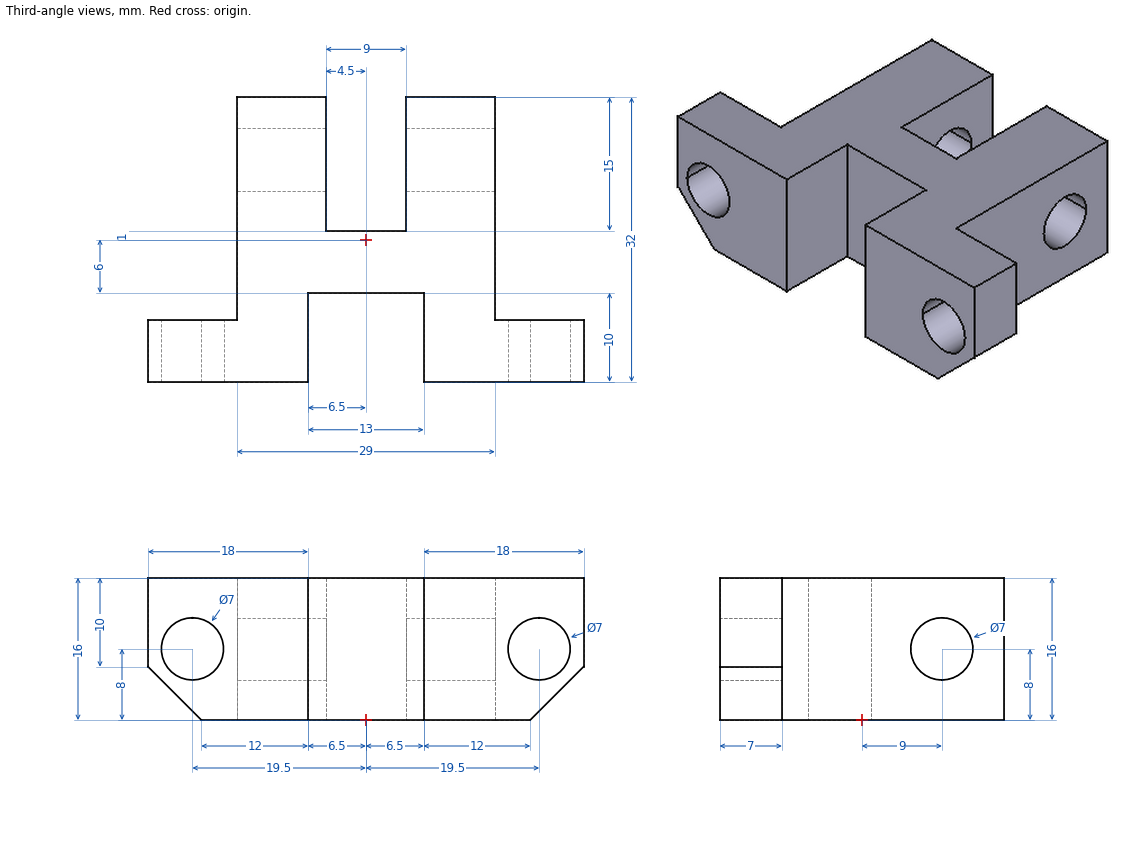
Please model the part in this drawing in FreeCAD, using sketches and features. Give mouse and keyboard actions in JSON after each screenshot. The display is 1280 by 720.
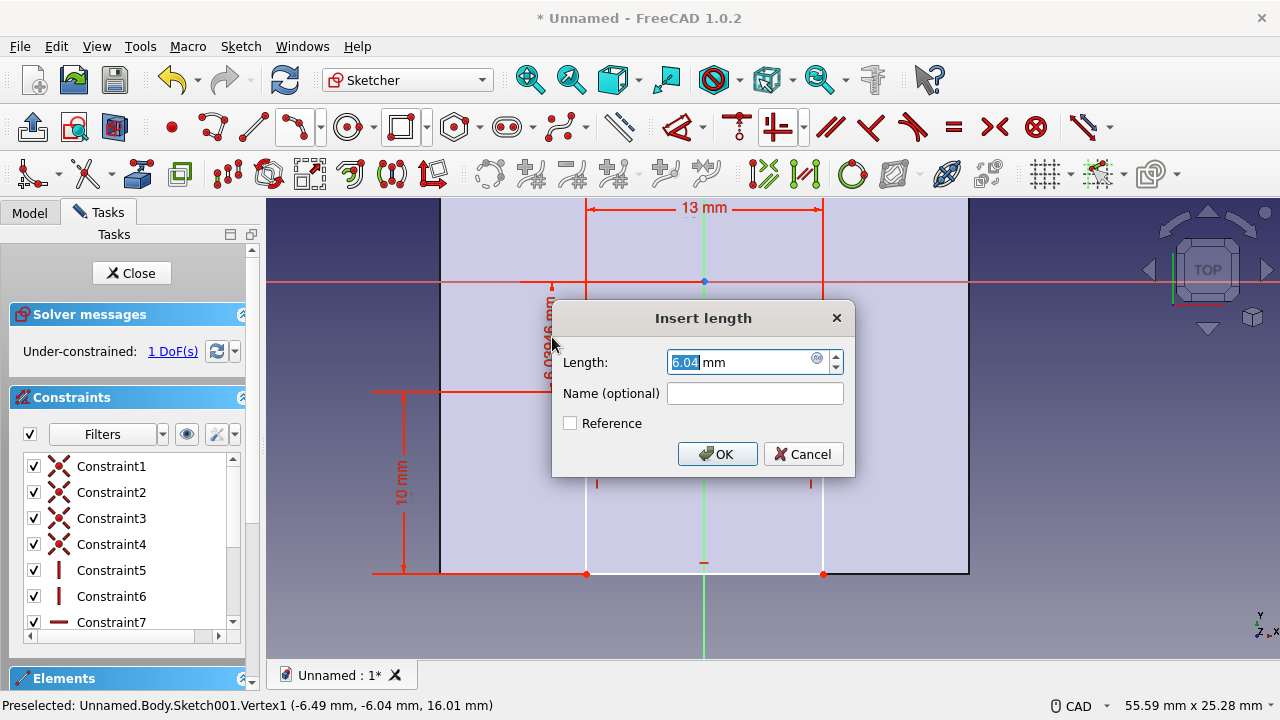
{"action": "type", "text": "6"}
{"action": "key", "text": "Return"}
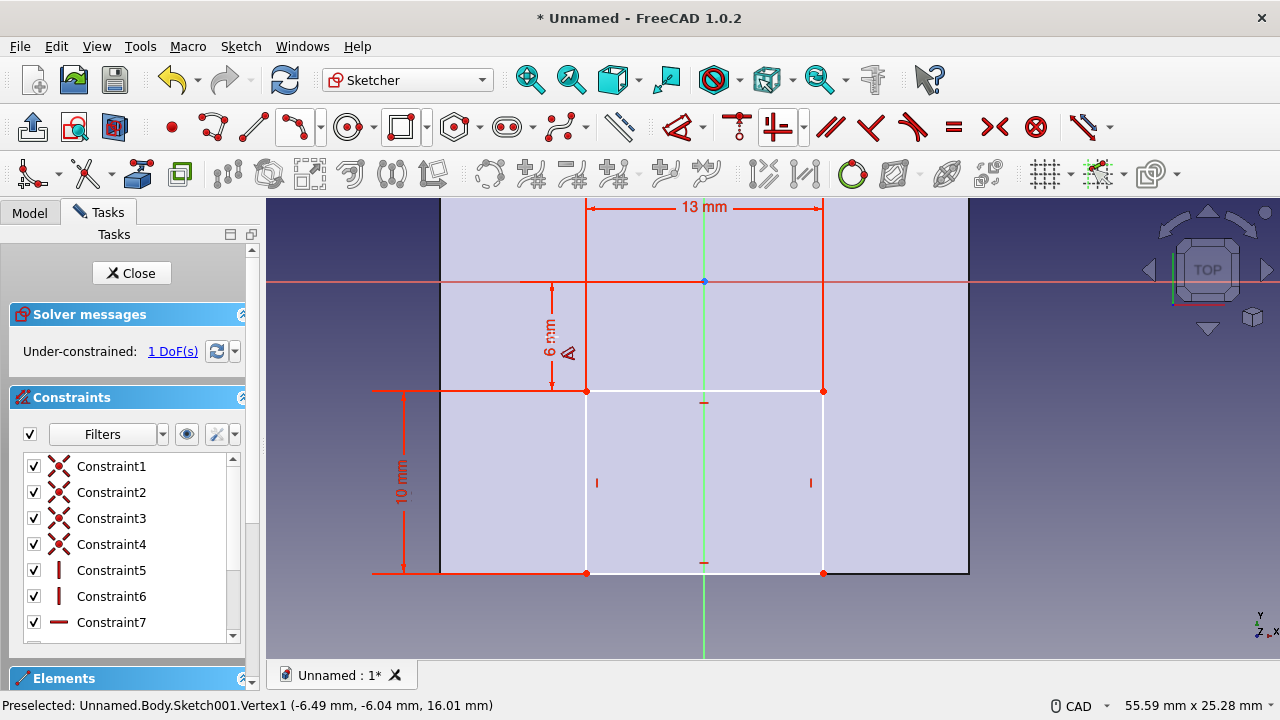
{"action": "left_click", "coordinate": [586, 391]}
{"action": "left_click", "coordinate": [645, 248]}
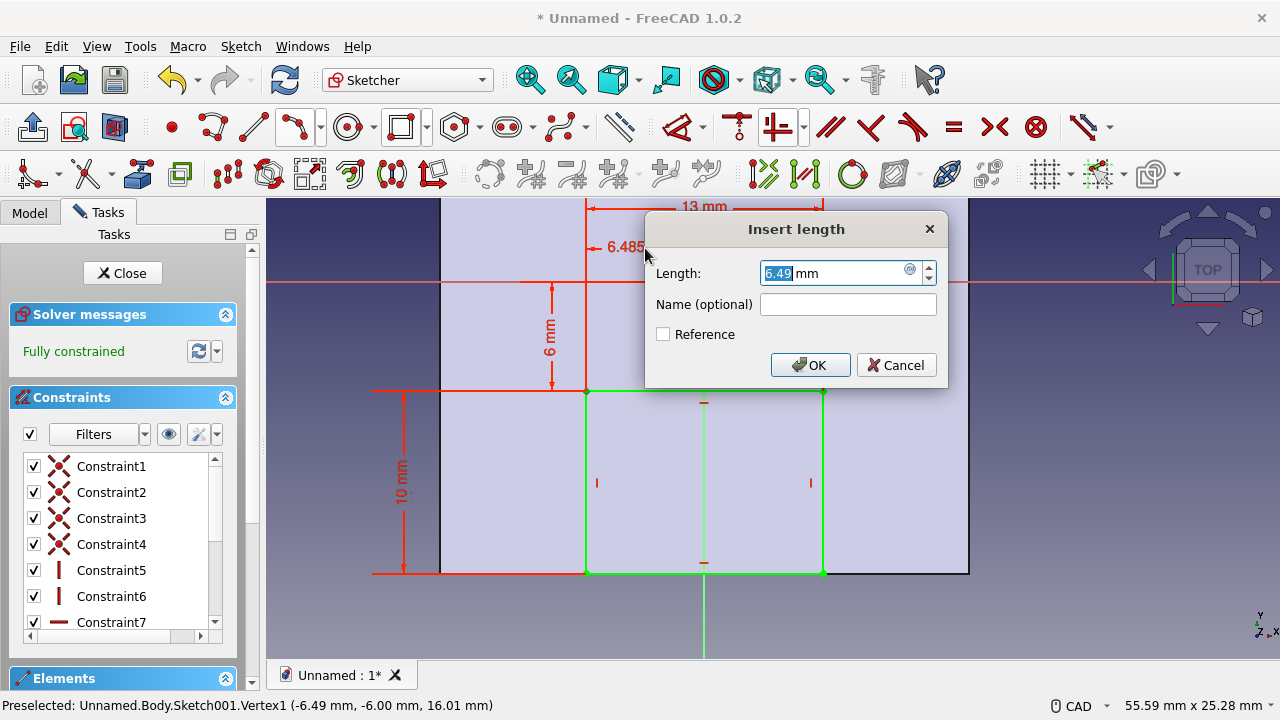
{"action": "type", "text": "6.5"}
{"action": "key", "text": "Return"}
{"action": "key", "text": "Escape"}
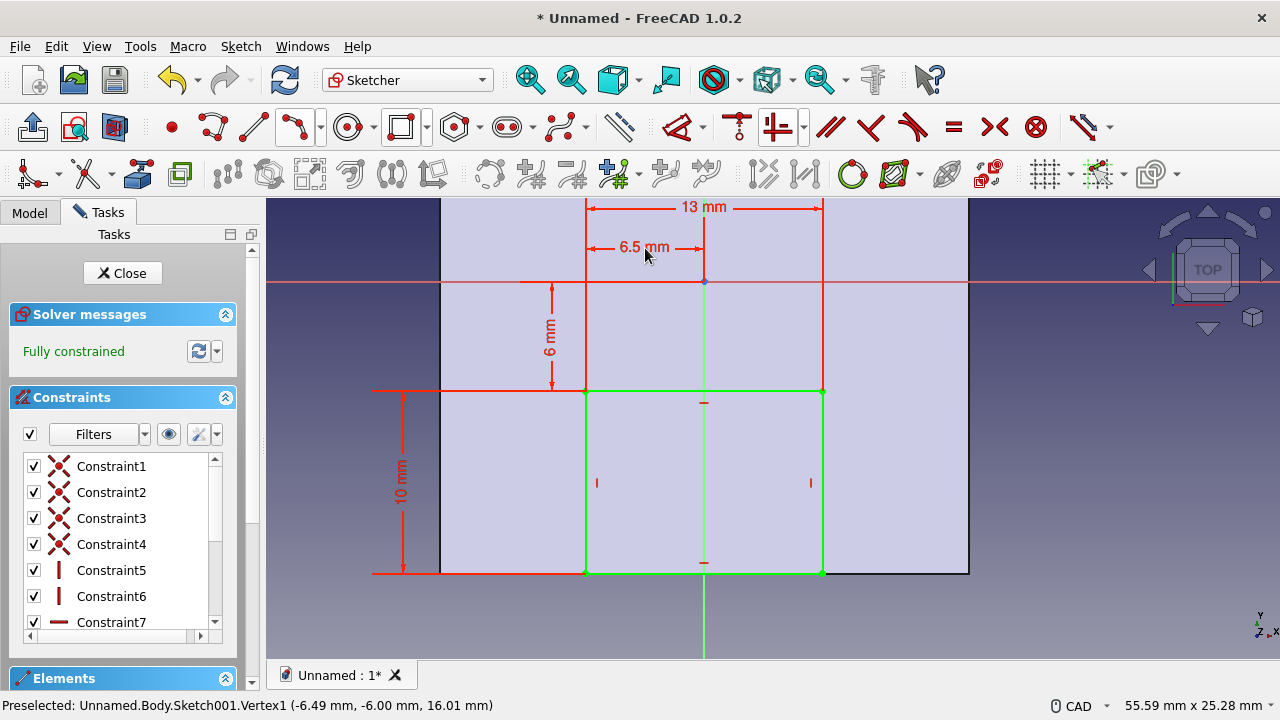
{"action": "left_click", "coordinate": [123, 273]}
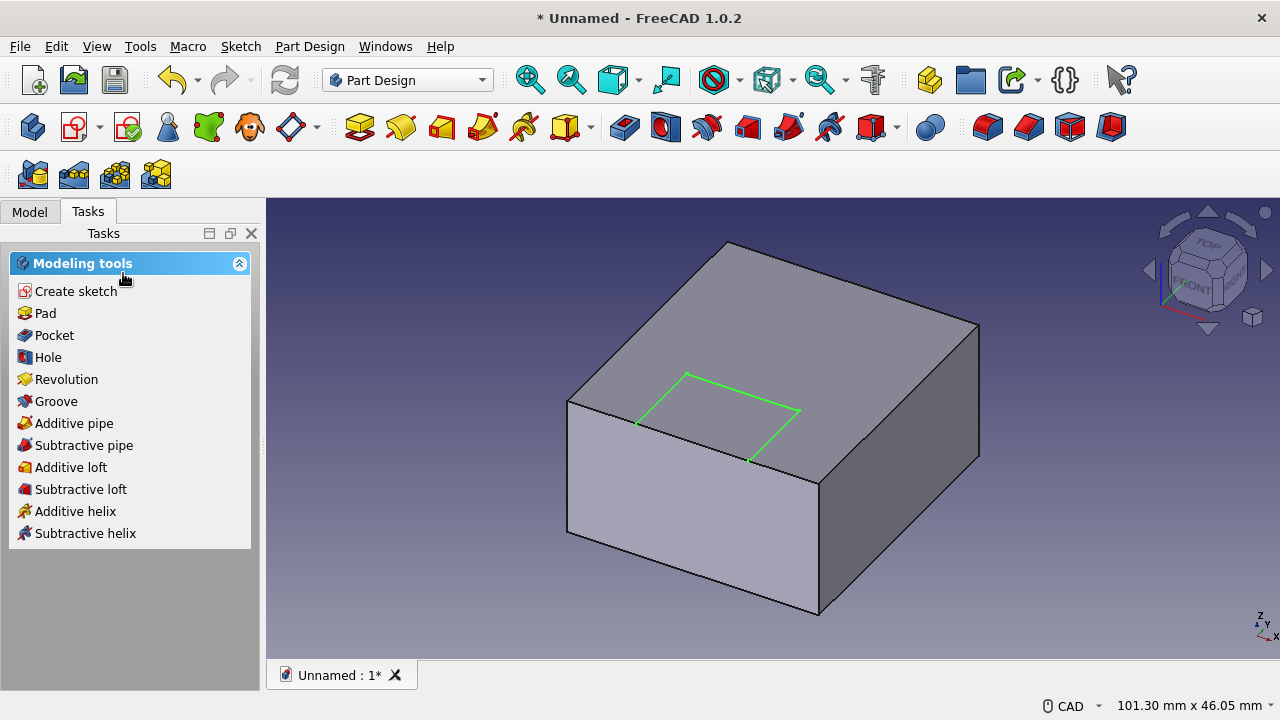
{"action": "left_click", "coordinate": [625, 128]}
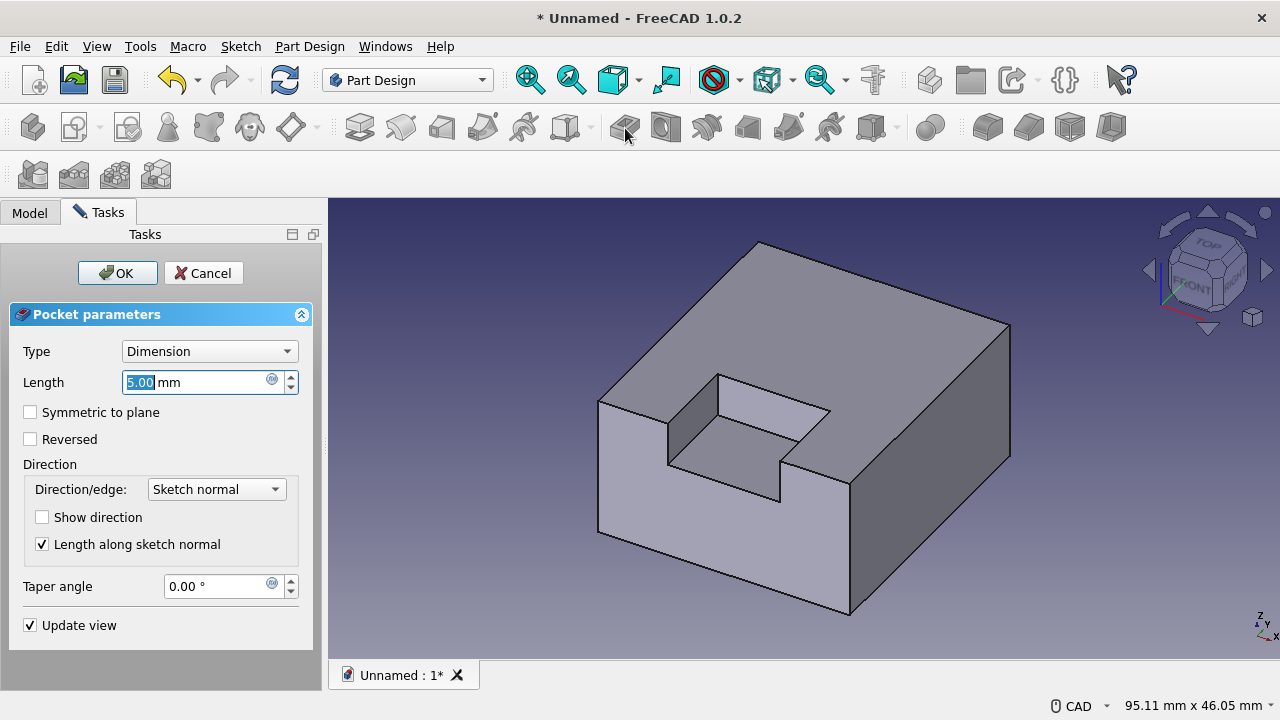
{"action": "type", "text": "16"}
{"action": "key", "text": "Tab"}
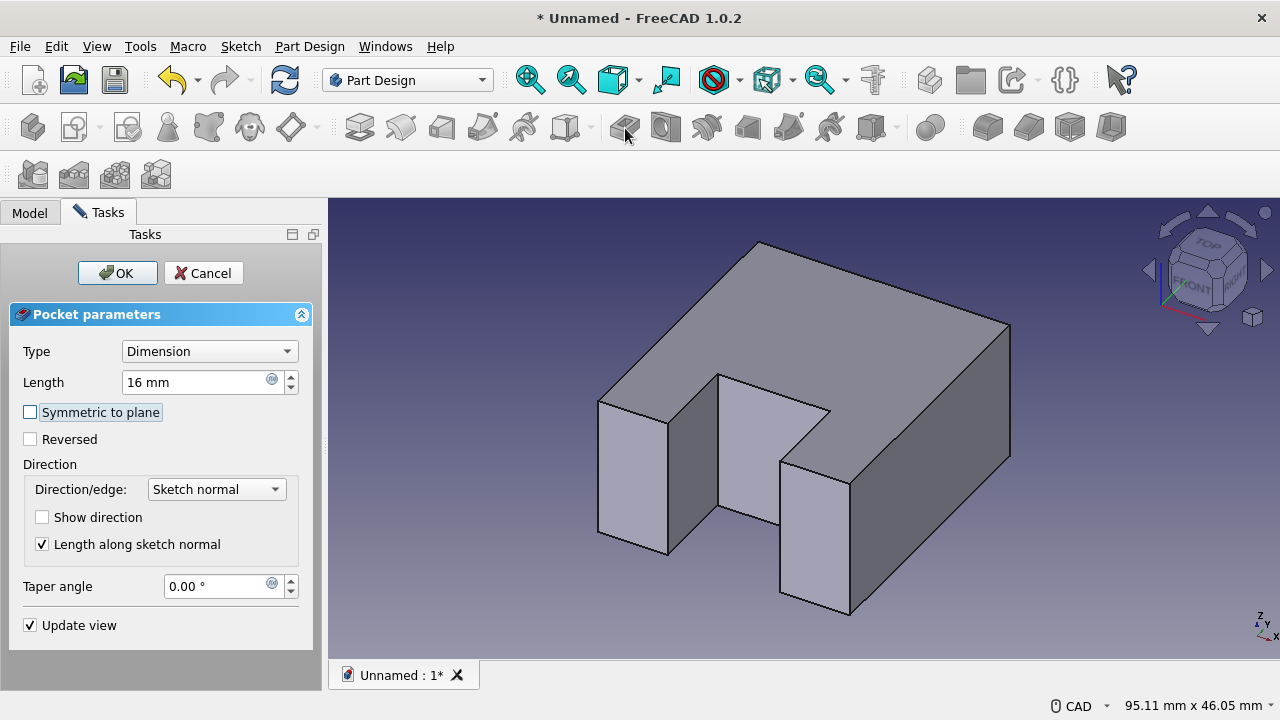
{"action": "left_click", "coordinate": [118, 273]}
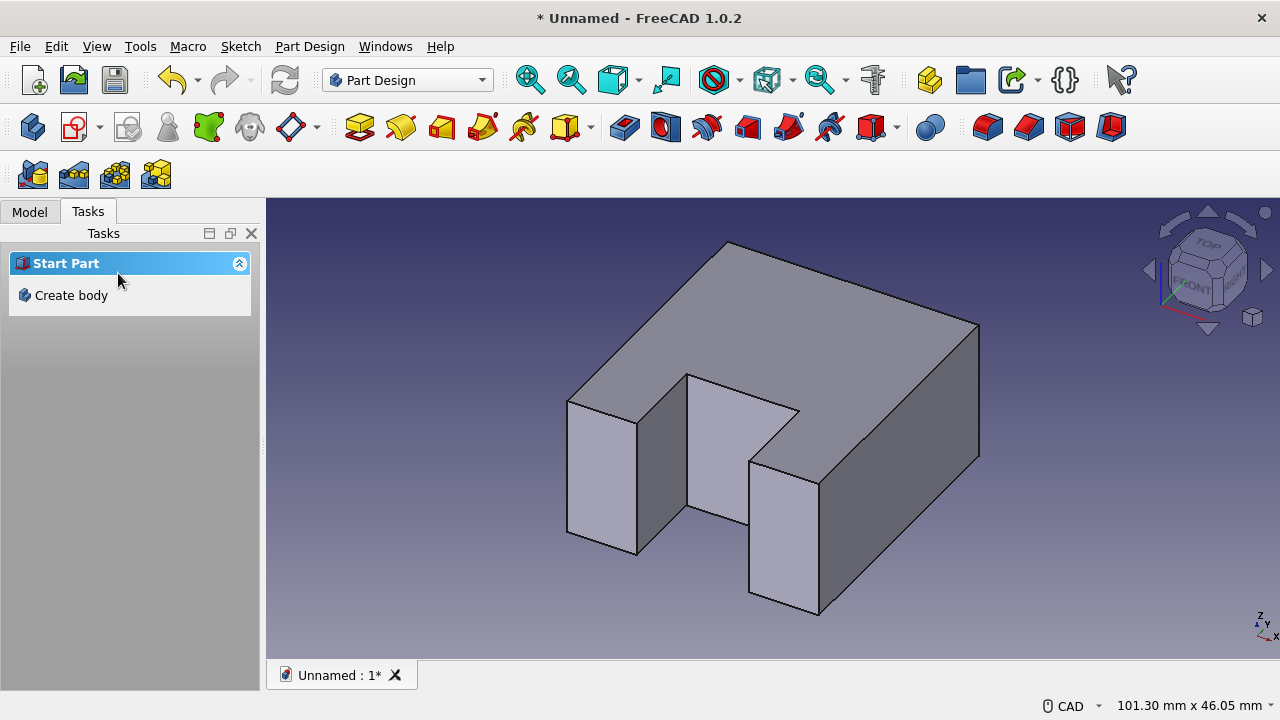
{"action": "left_click", "coordinate": [796, 339]}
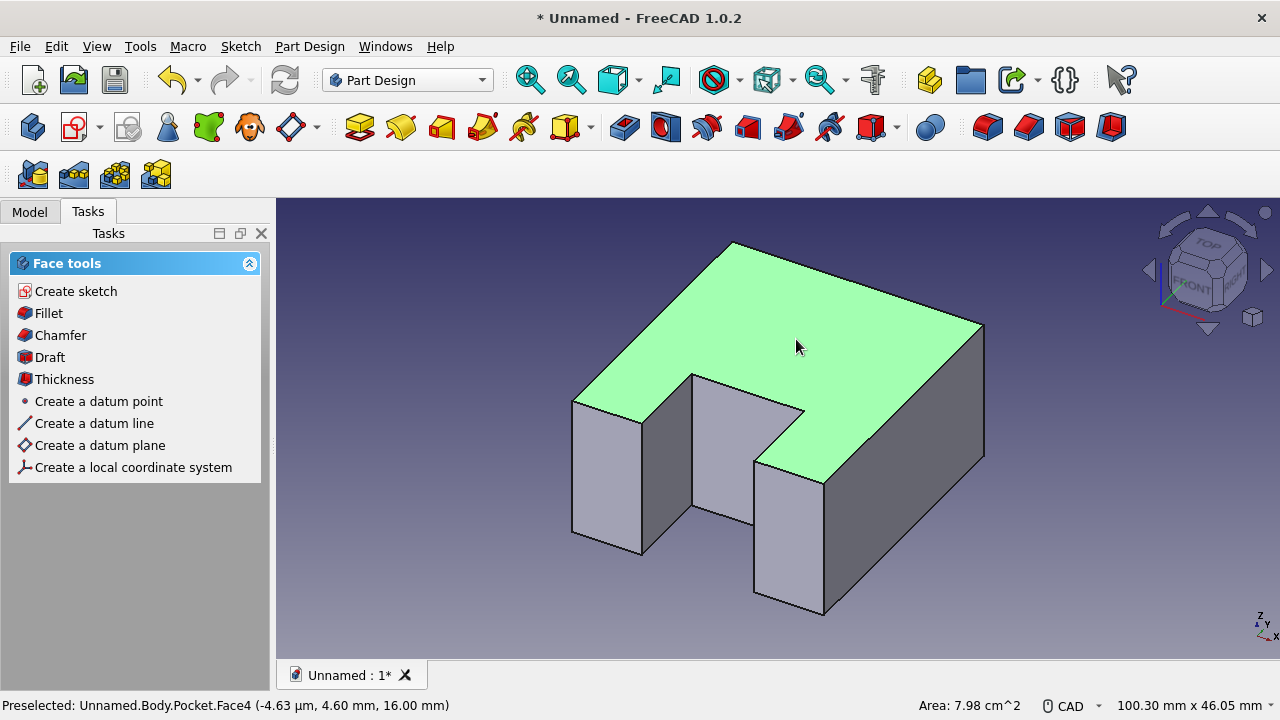
{"action": "left_click", "coordinate": [74, 128]}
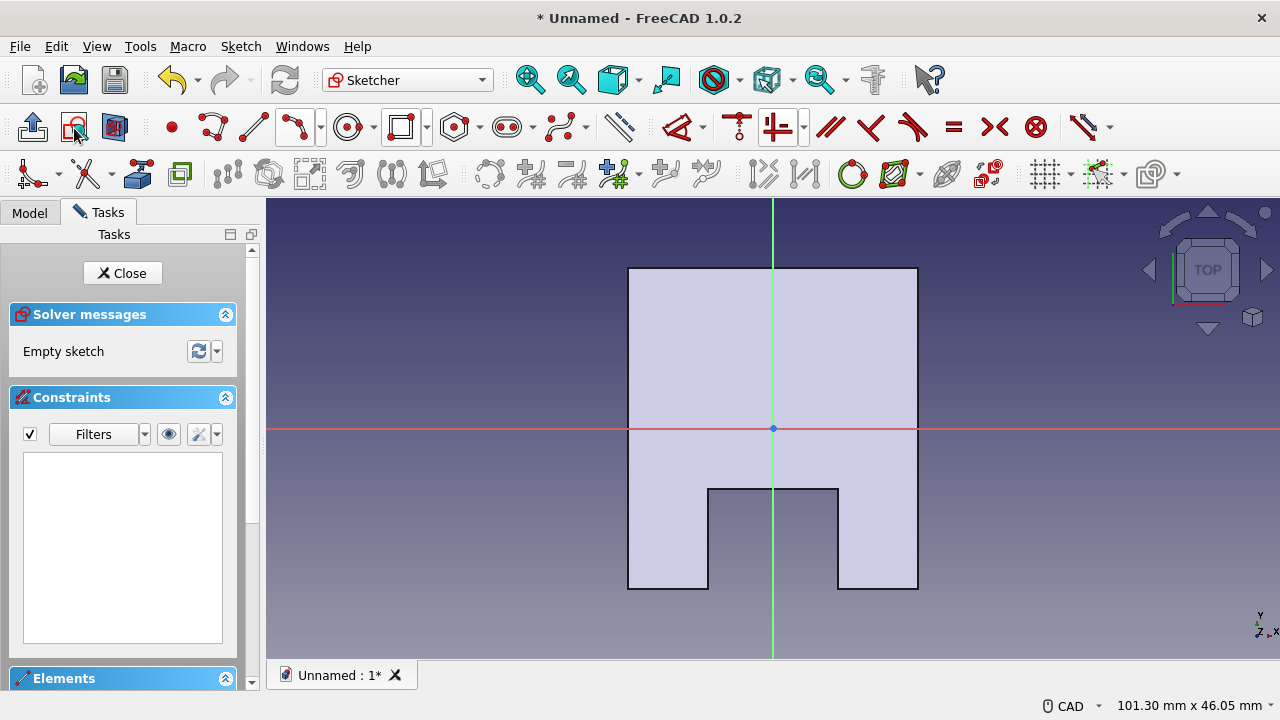
{"action": "scroll", "coordinate": [856, 251], "scroll_direction": "up", "scroll_amount": 3}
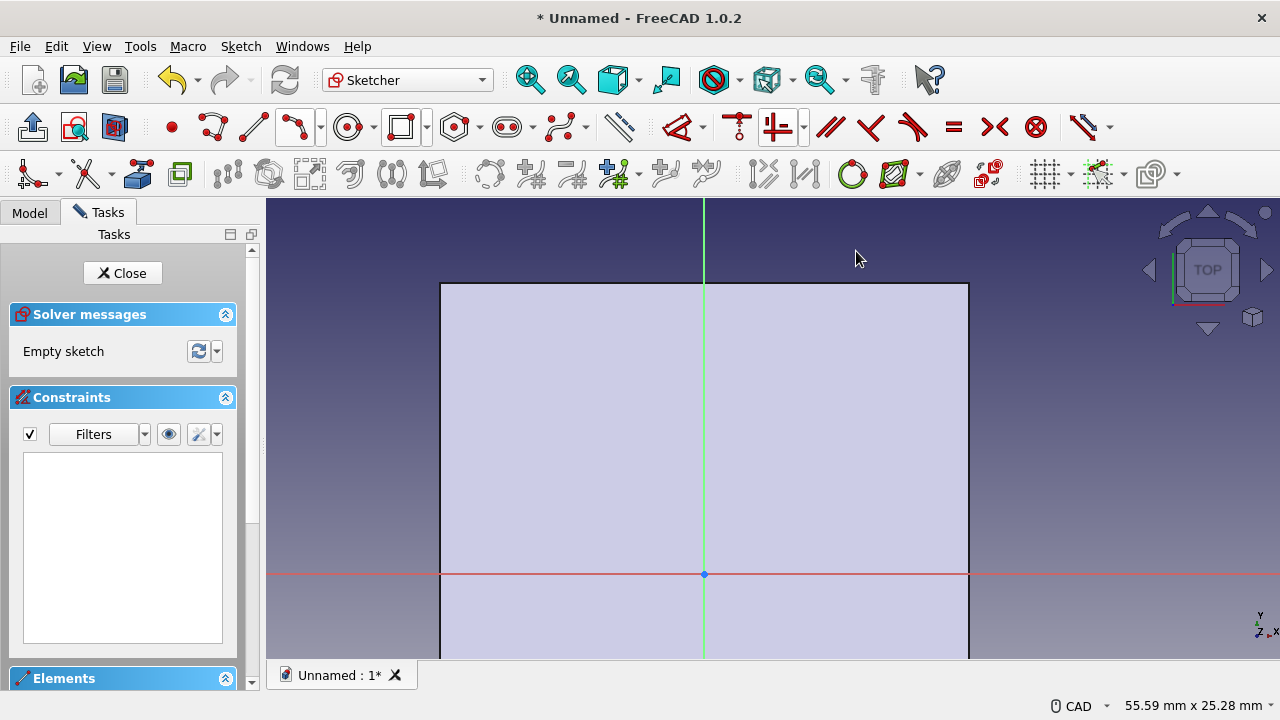
{"action": "left_click", "coordinate": [400, 128]}